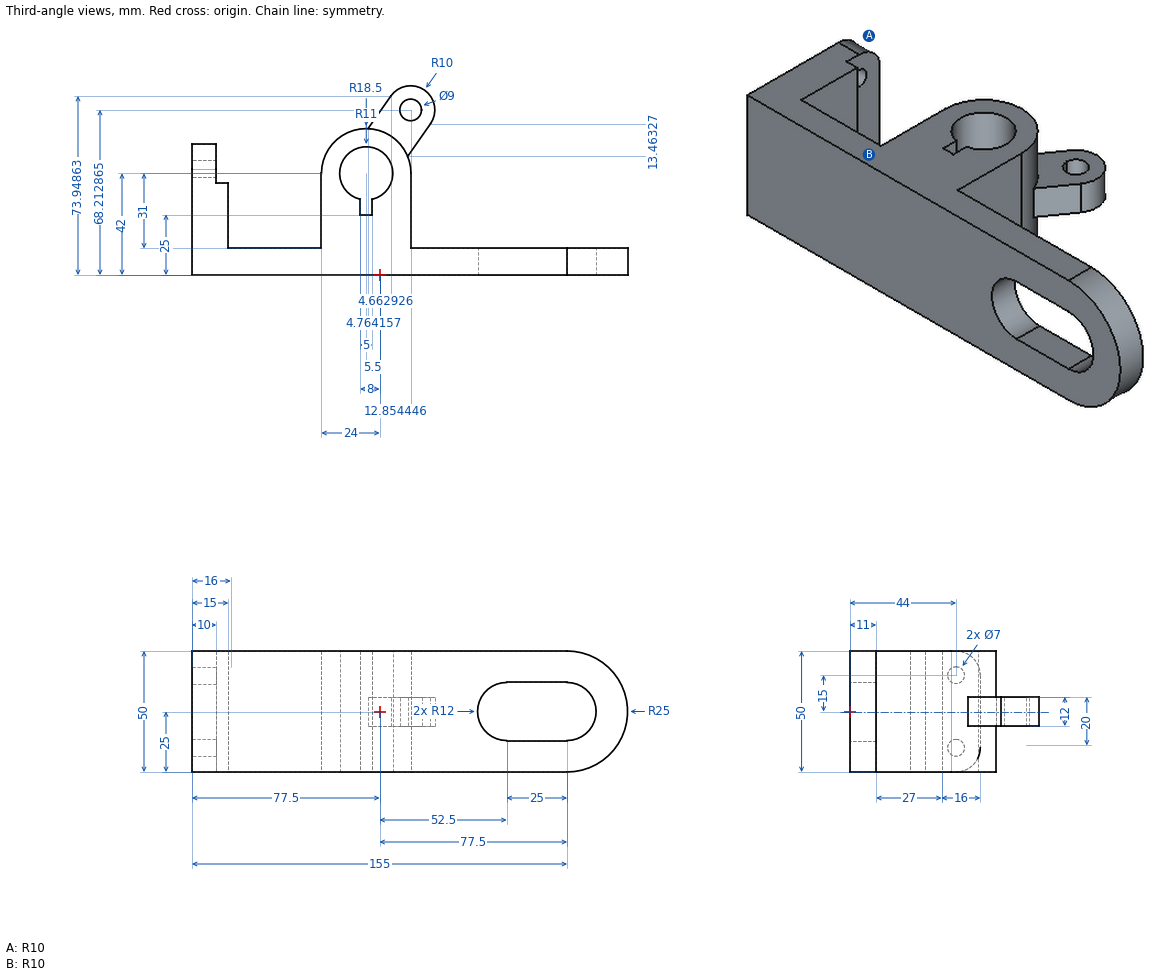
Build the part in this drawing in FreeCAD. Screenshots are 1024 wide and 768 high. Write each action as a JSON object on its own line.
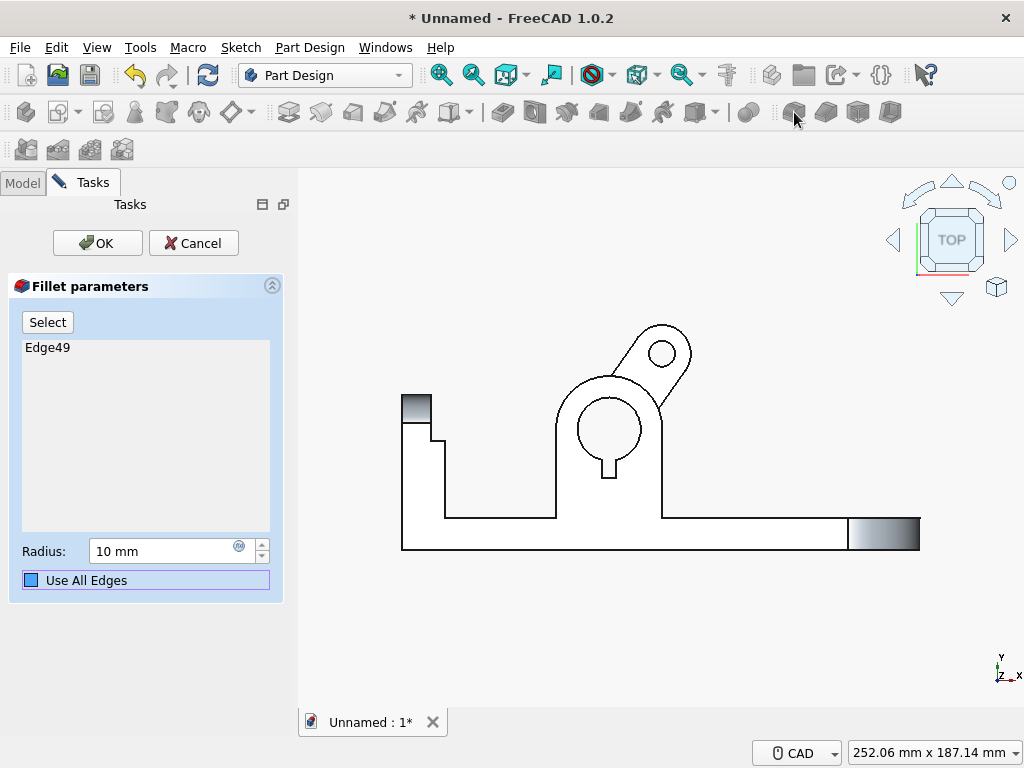
{"action": "left_click", "coordinate": [98, 243]}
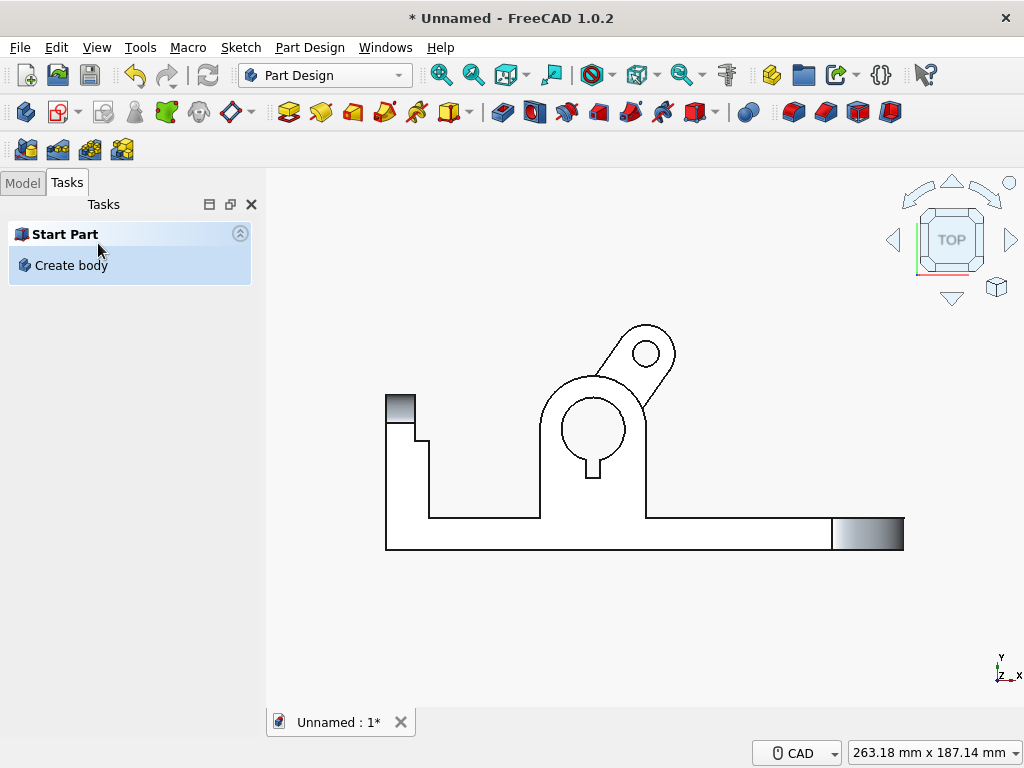
{"action": "key", "text": "0"}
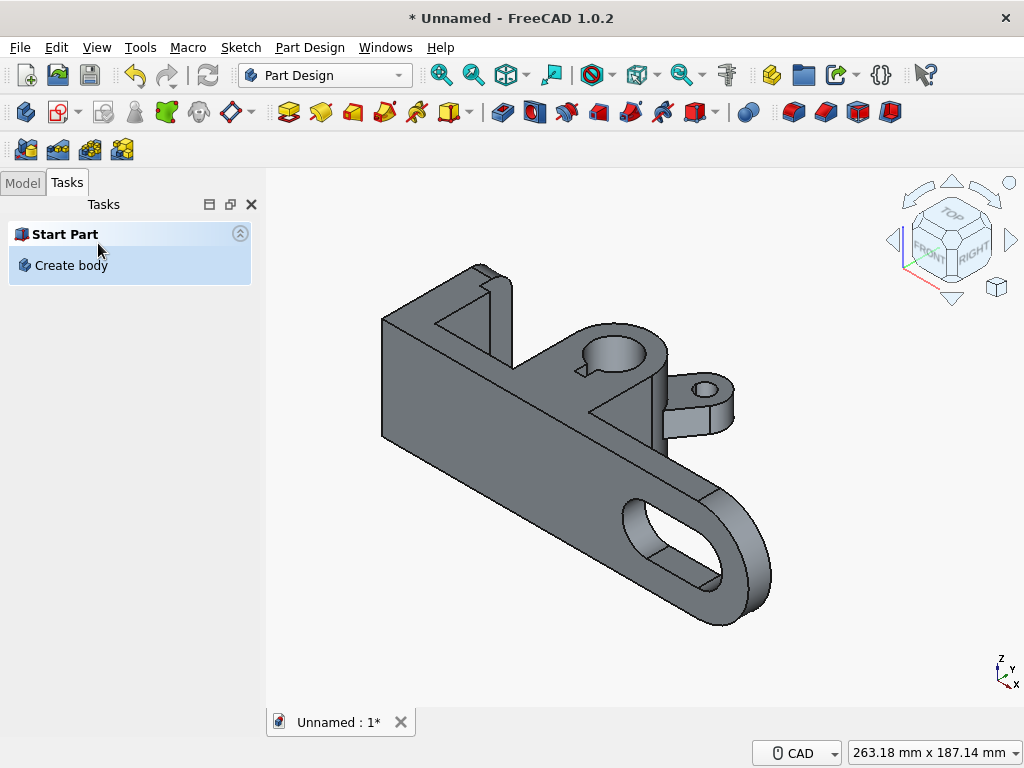
{"action": "key", "text": "2"}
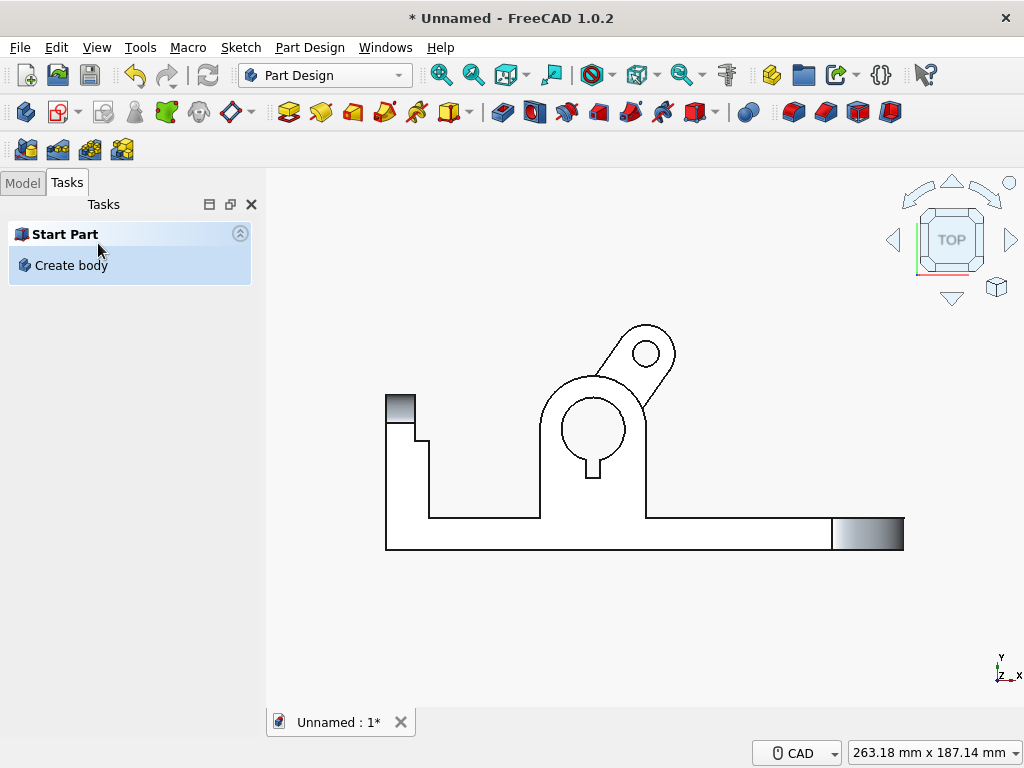
{"action": "key", "text": "1"}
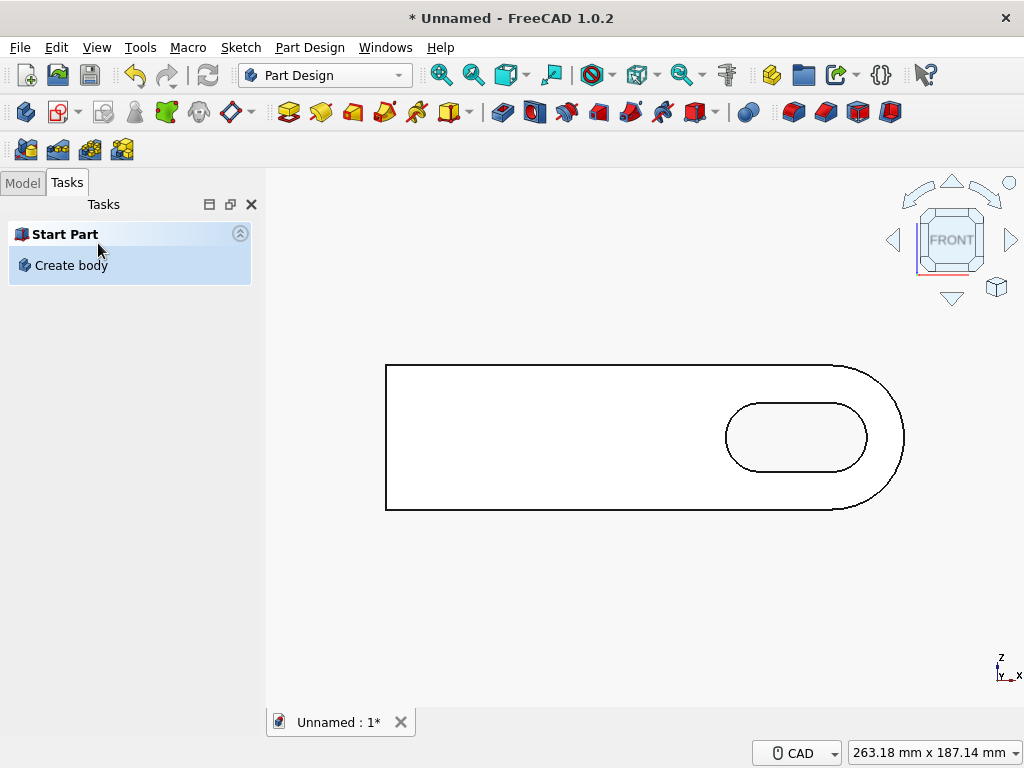
{"action": "key", "text": "3"}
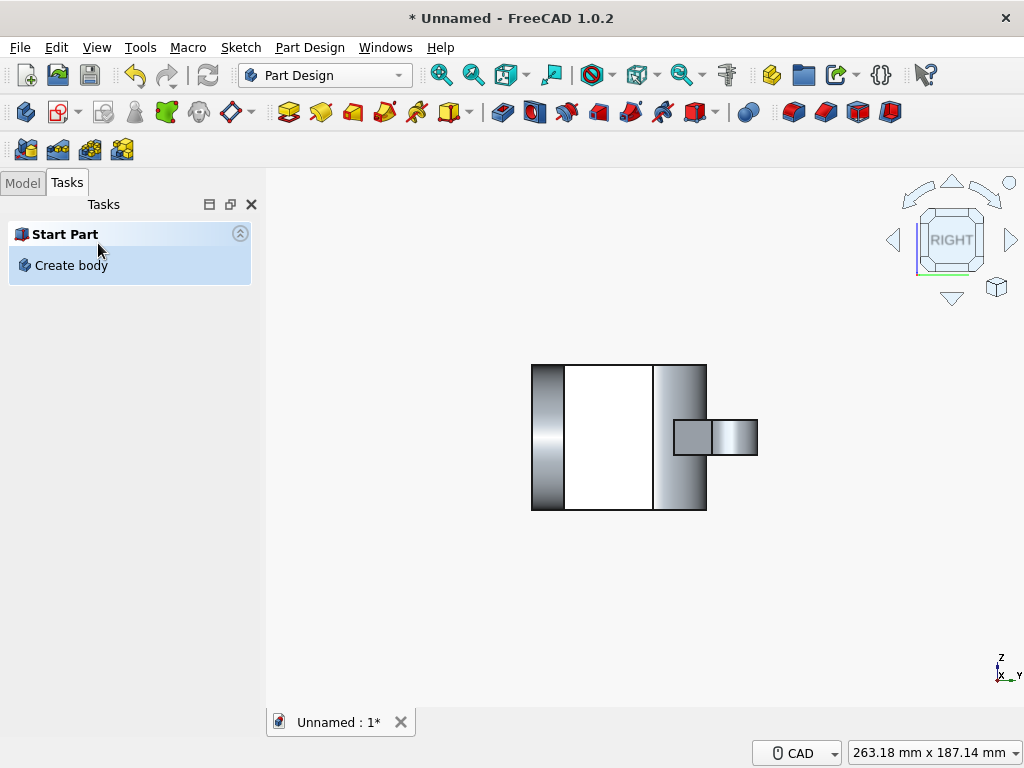
{"action": "left_click", "coordinate": [442, 76]}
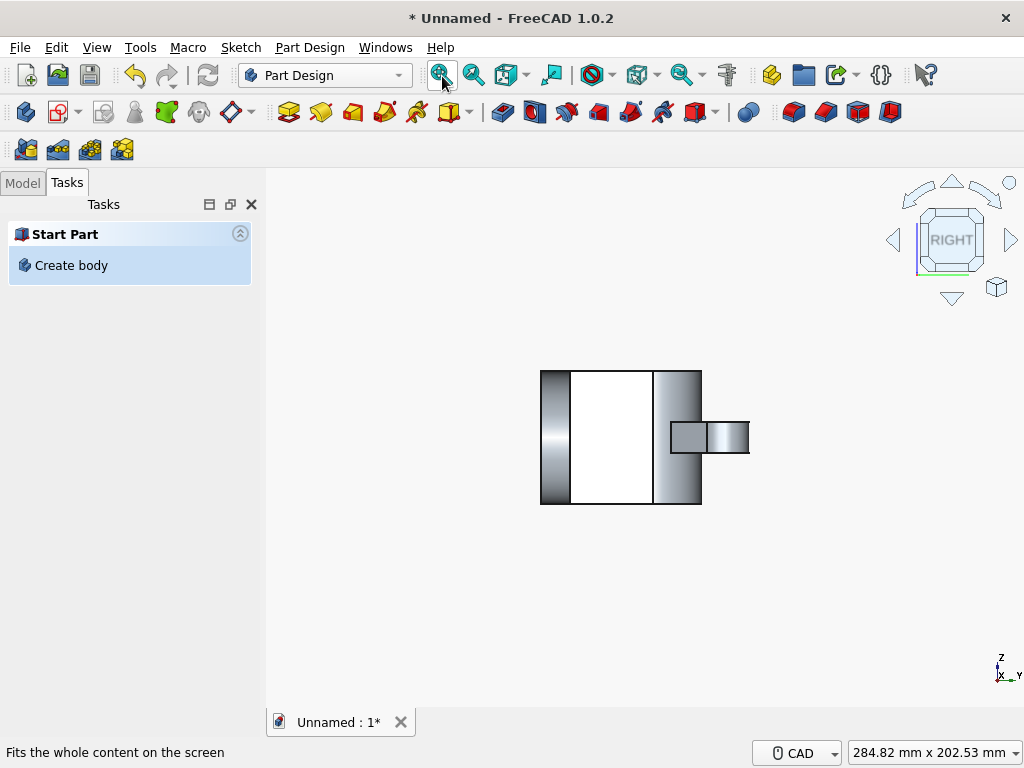
{"action": "key", "text": "5"}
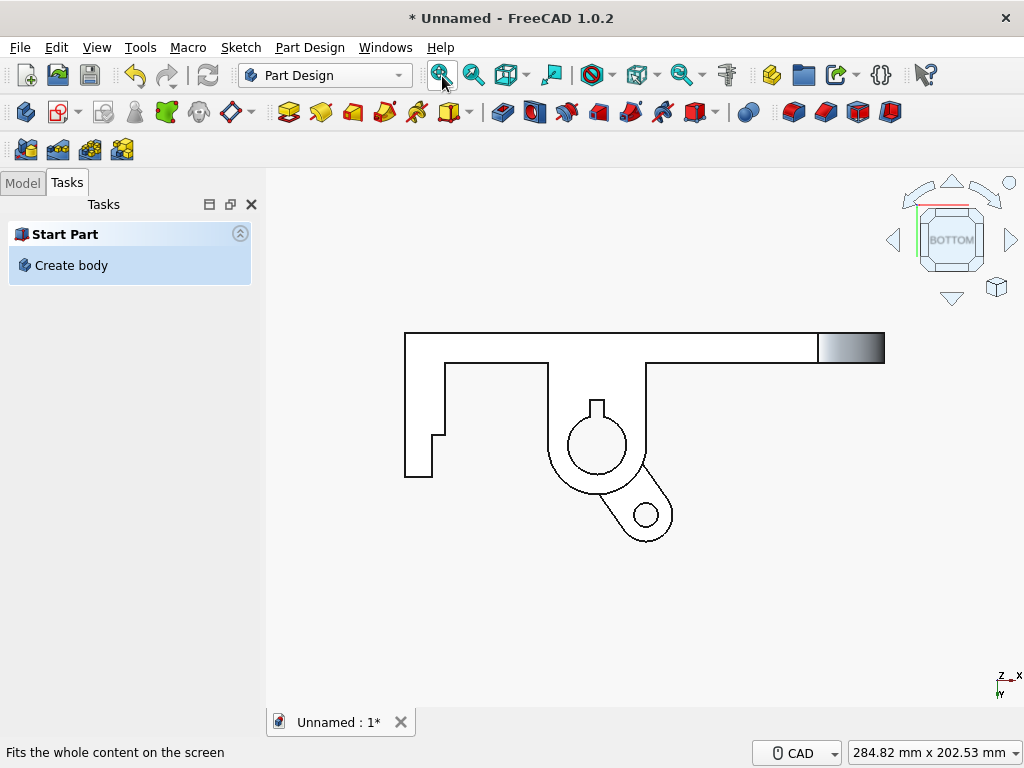
{"action": "key", "text": "4"}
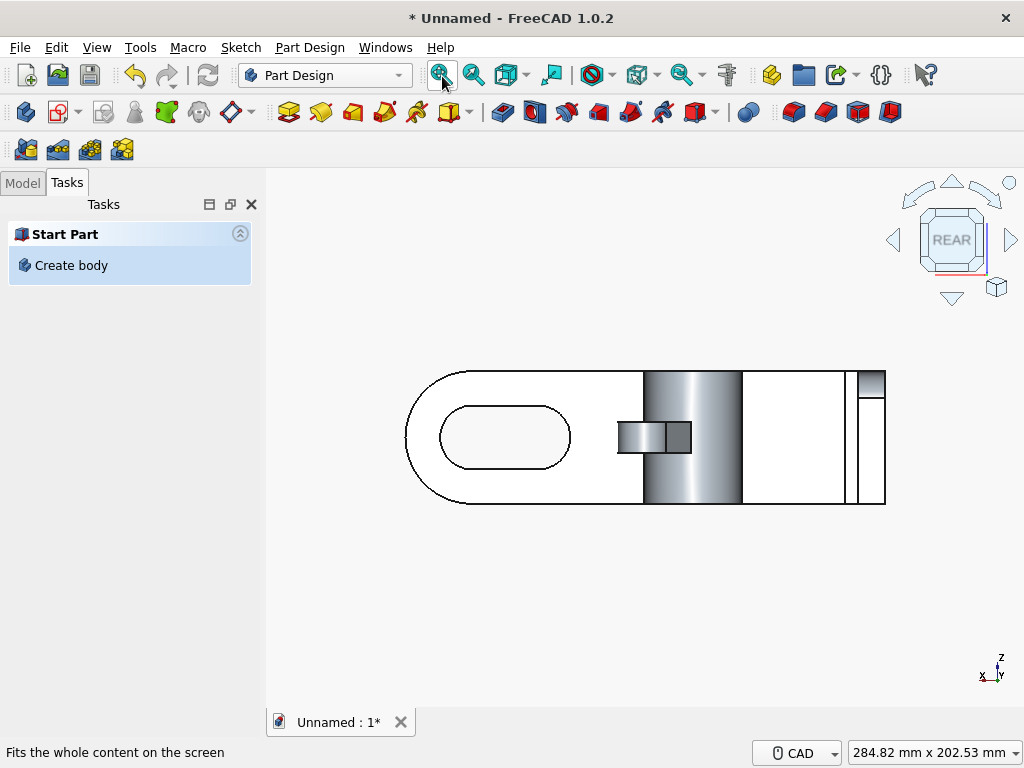
{"action": "left_click", "coordinate": [871, 503]}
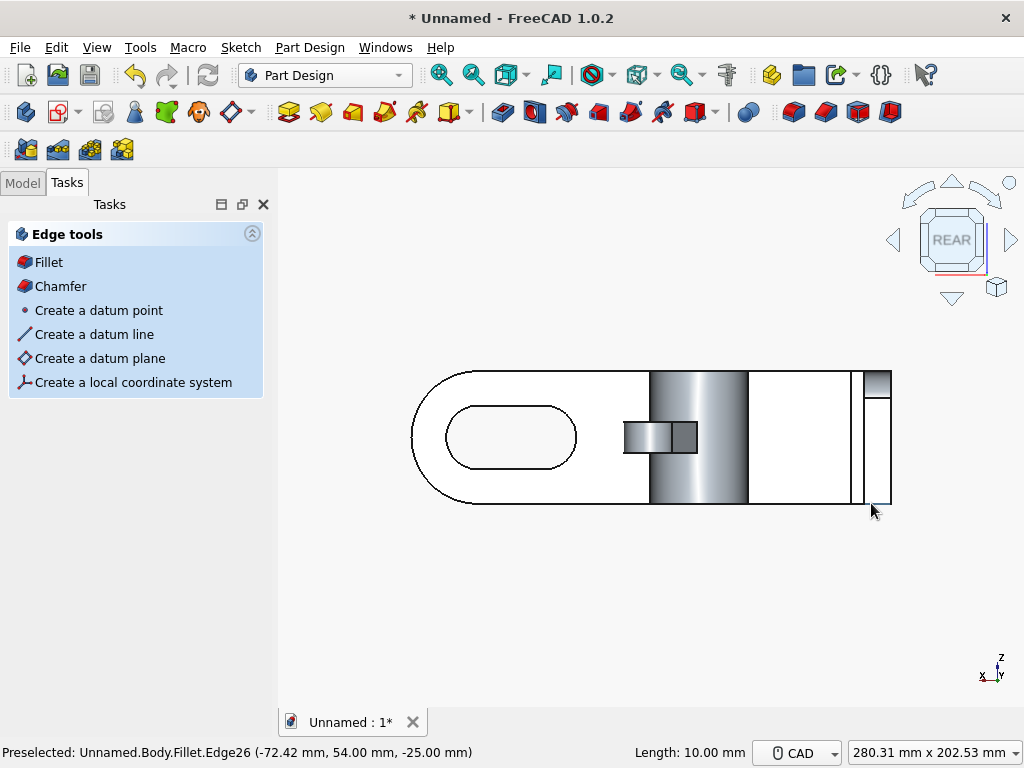
{"action": "left_click", "coordinate": [794, 112]}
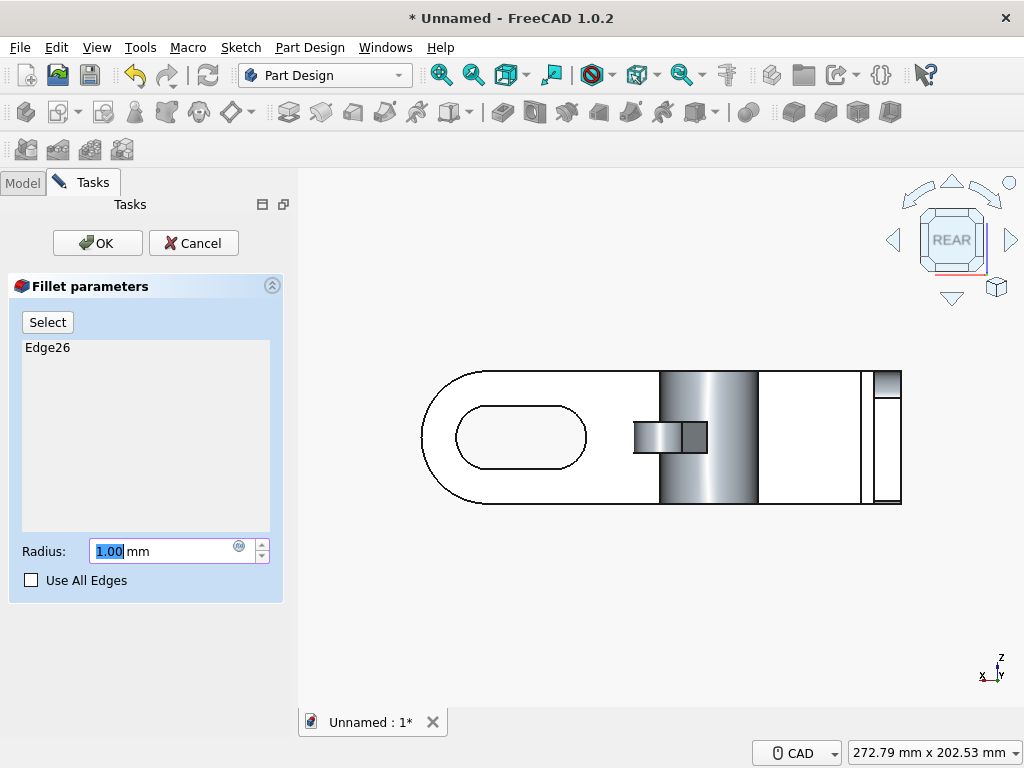
{"action": "type", "text": "10"}
{"action": "key", "text": "Tab"}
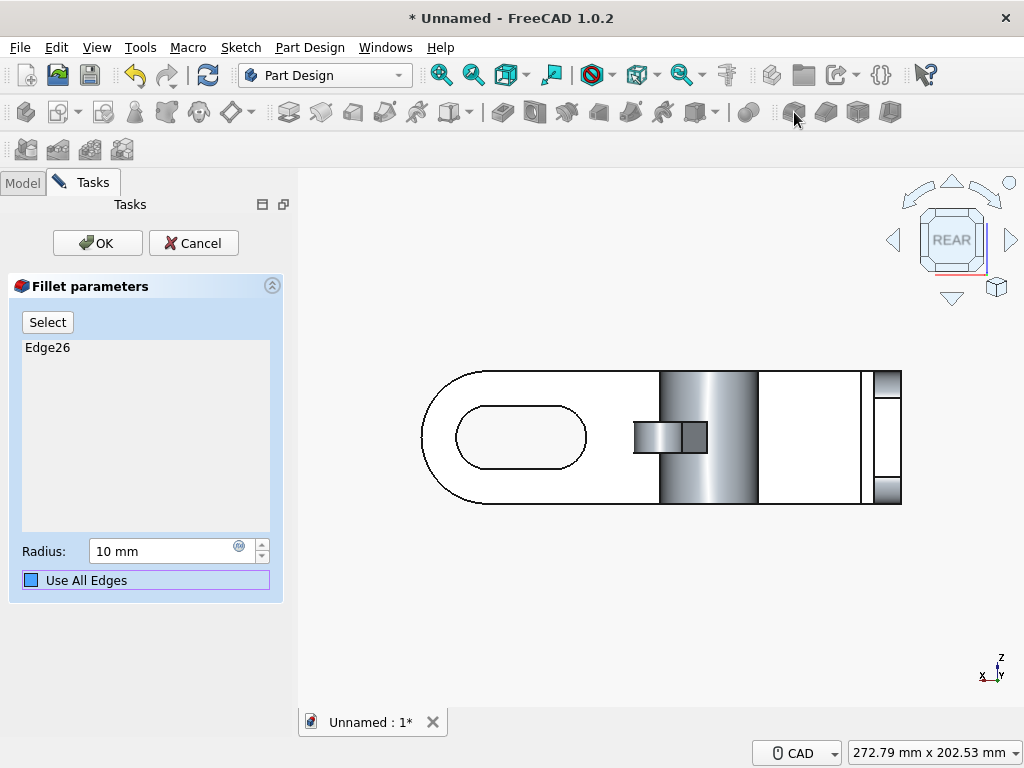
{"action": "left_click", "coordinate": [98, 243]}